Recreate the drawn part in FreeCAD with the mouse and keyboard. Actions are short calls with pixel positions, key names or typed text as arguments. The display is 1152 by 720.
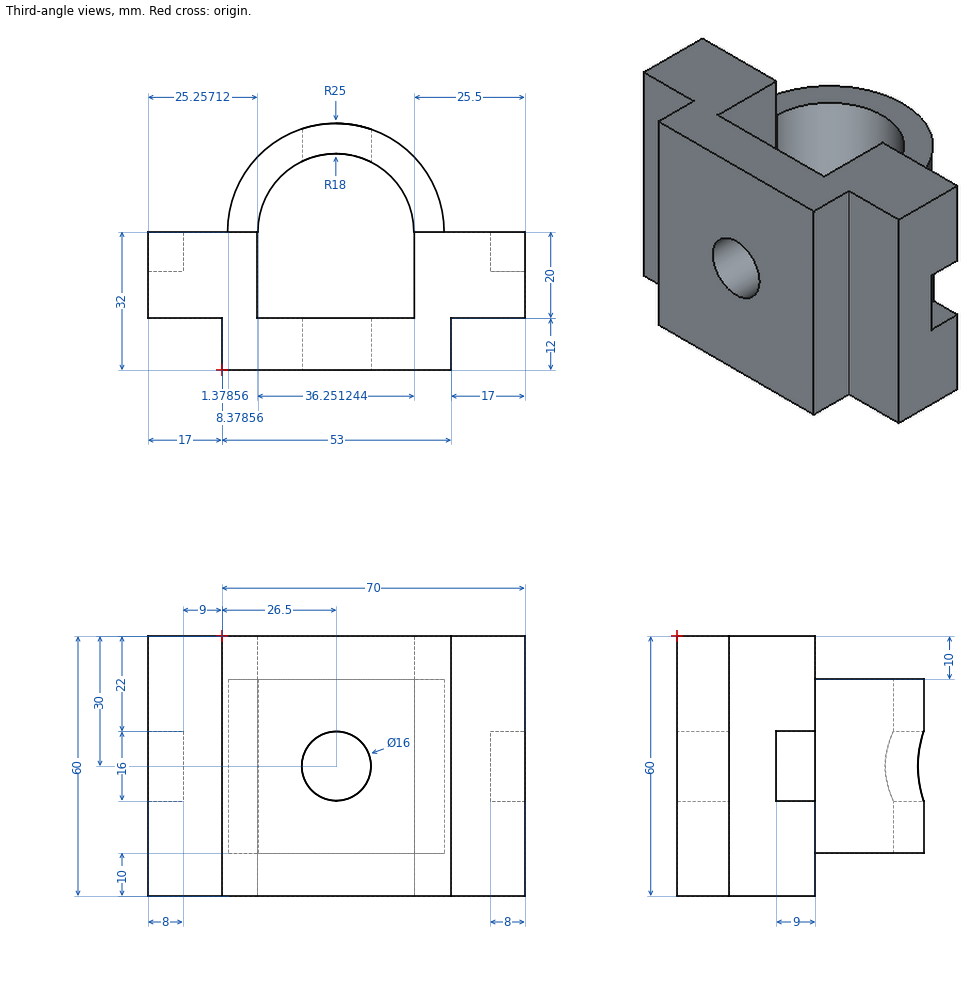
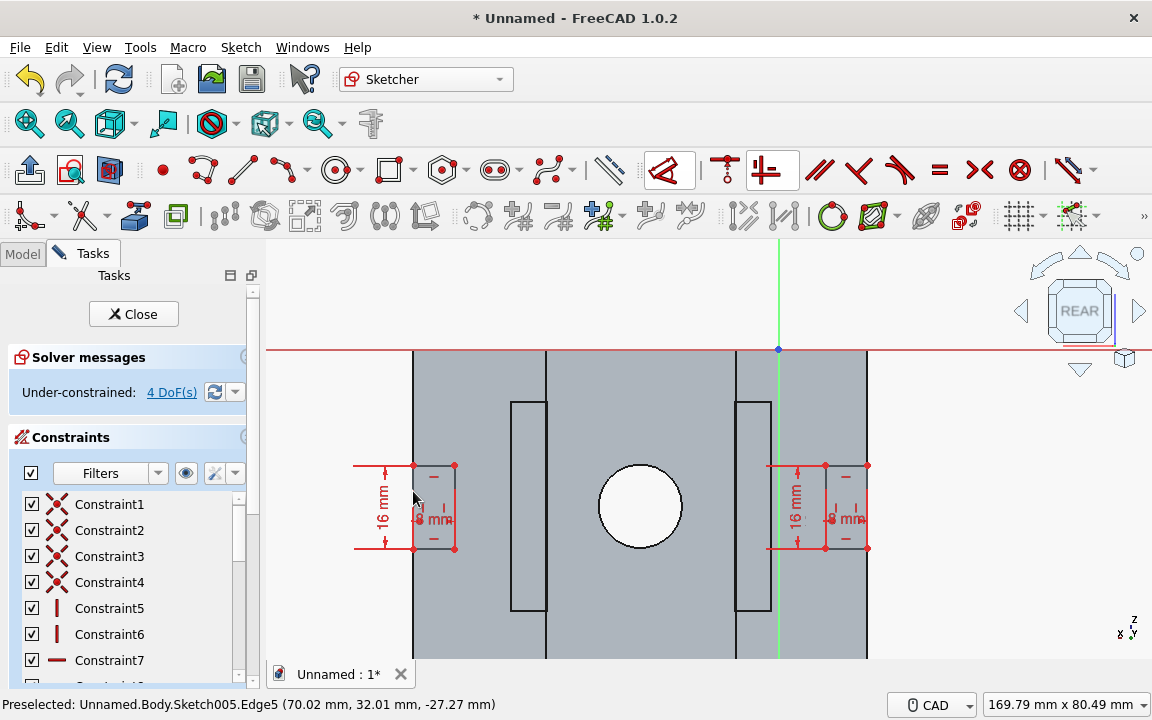
click(826, 466)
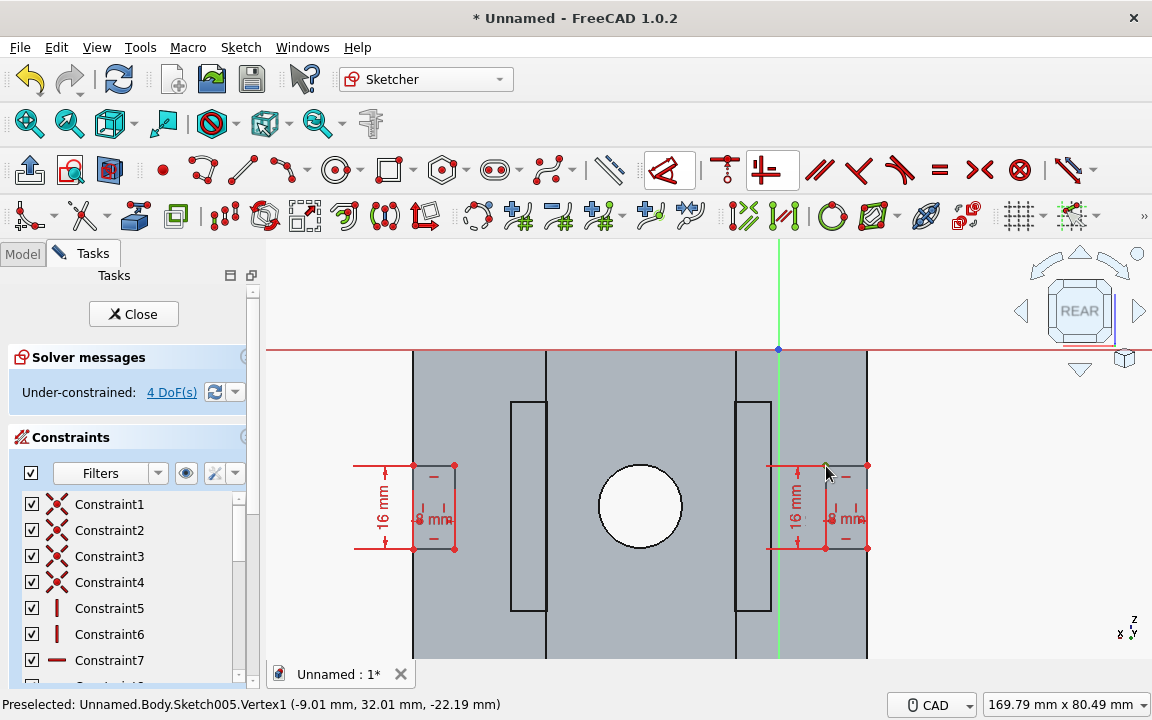
click(690, 170)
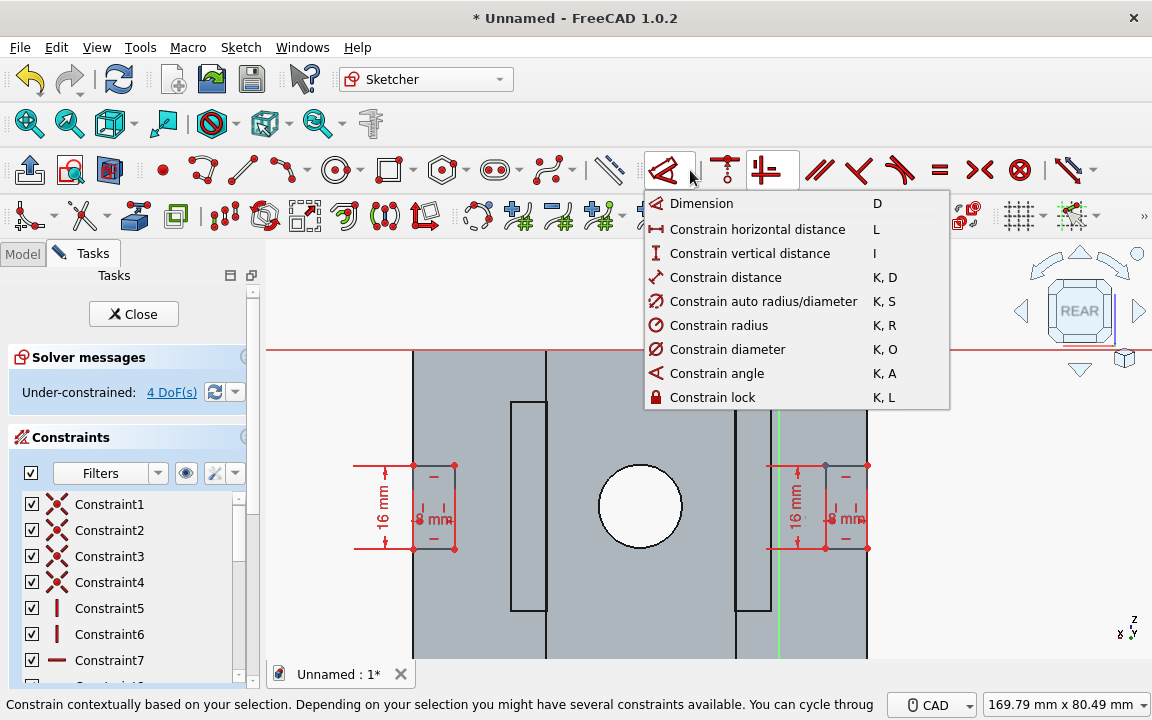
click(797, 229)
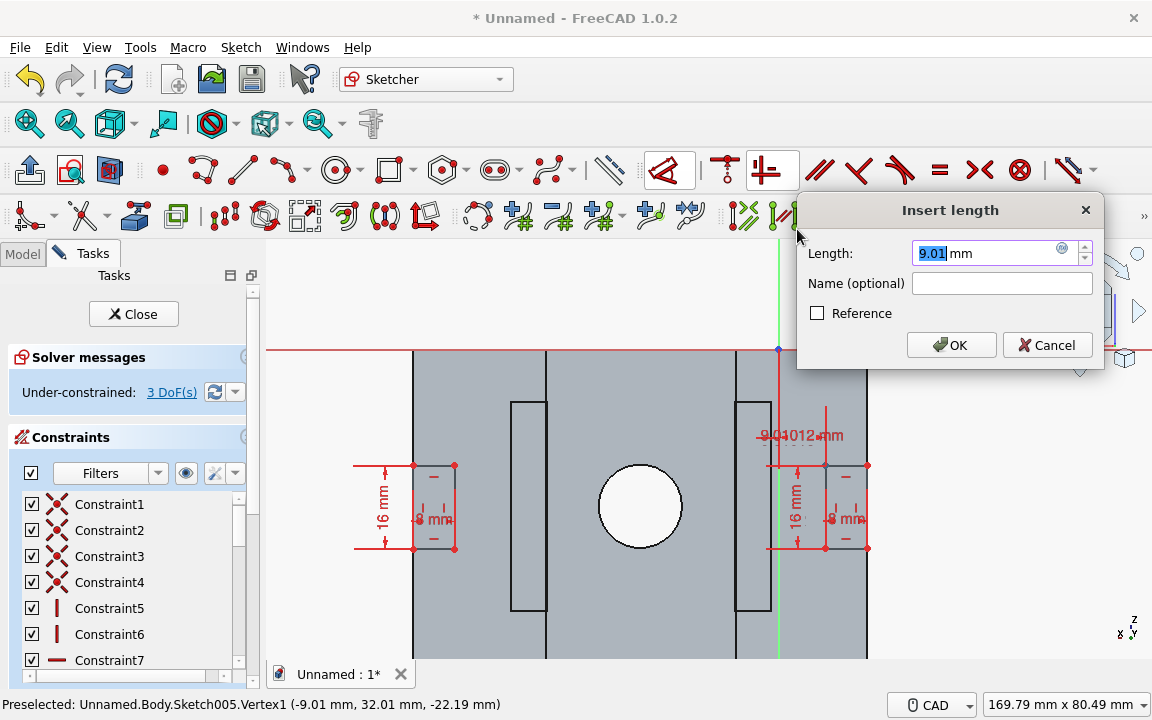
text(9)
key(Return)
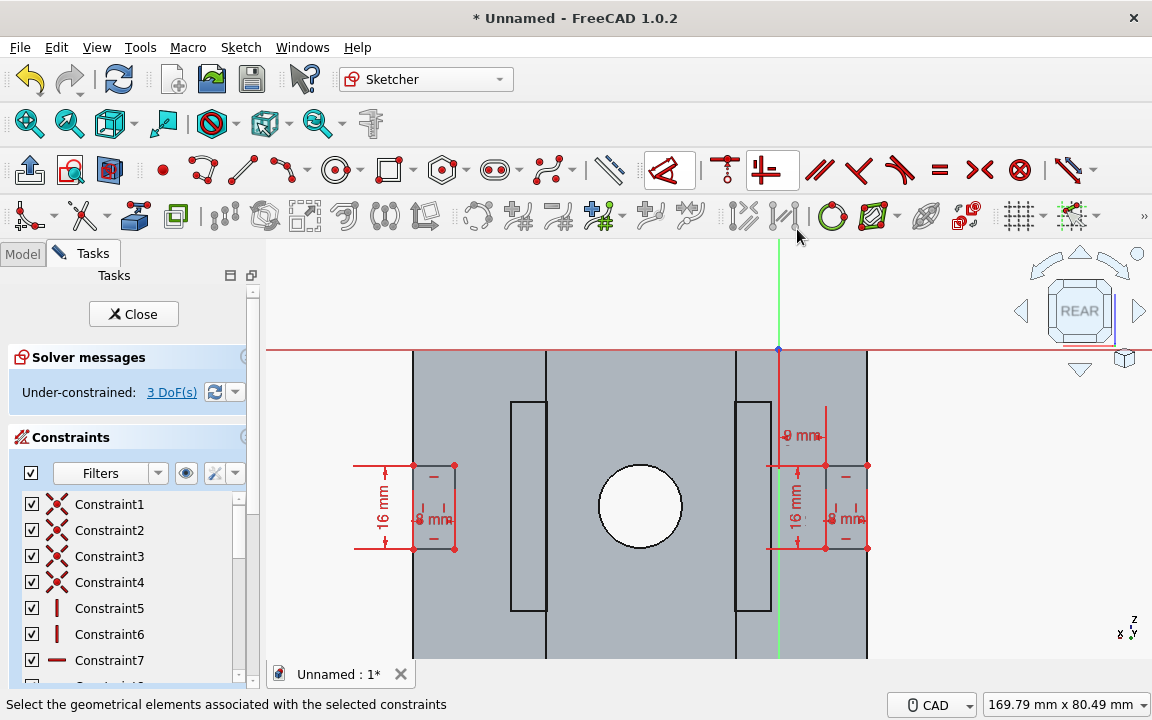
click(826, 466)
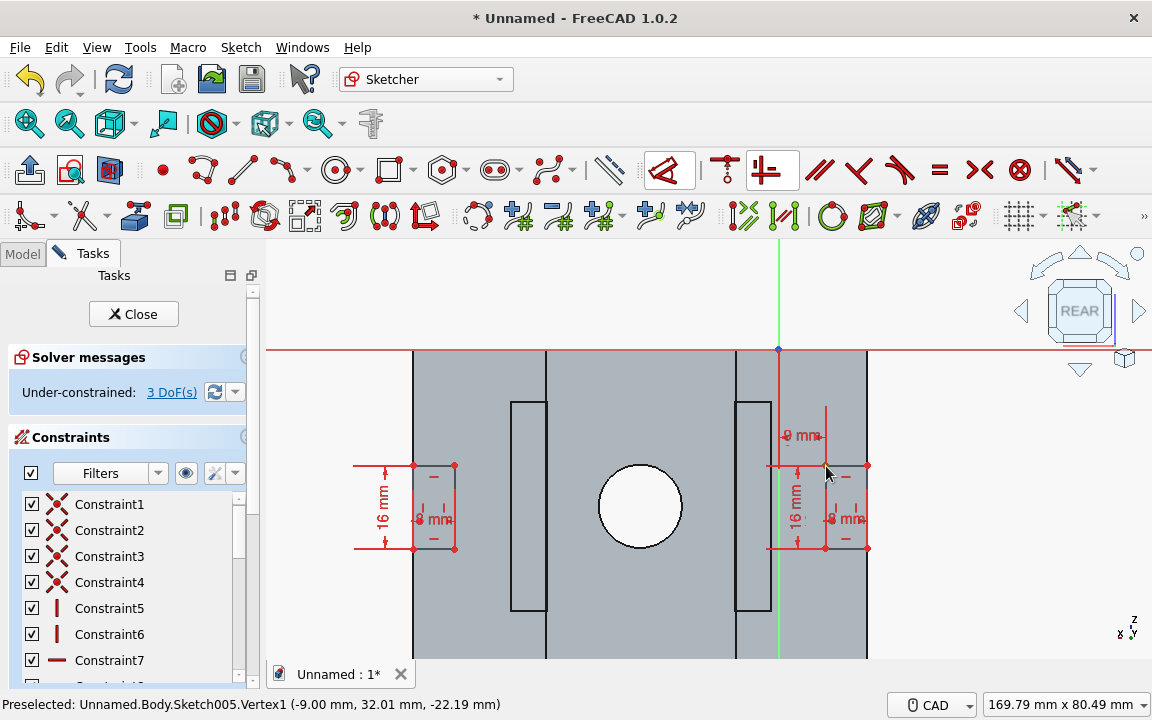
key(i)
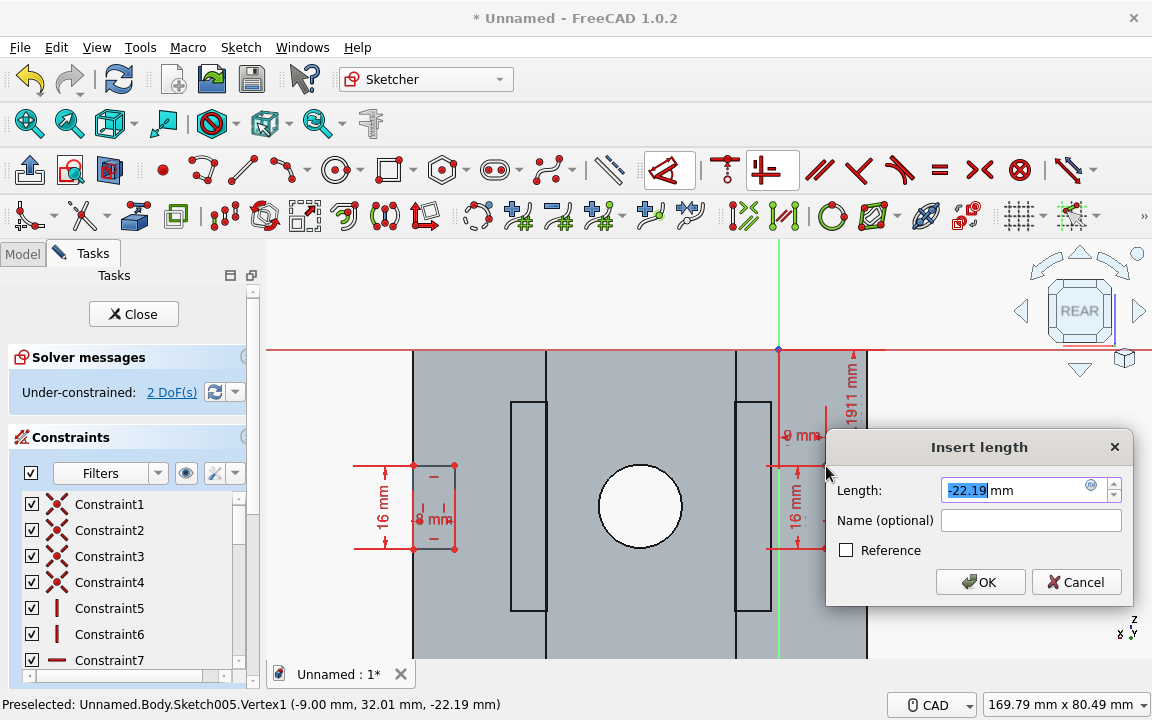
text(-22)
key(Return)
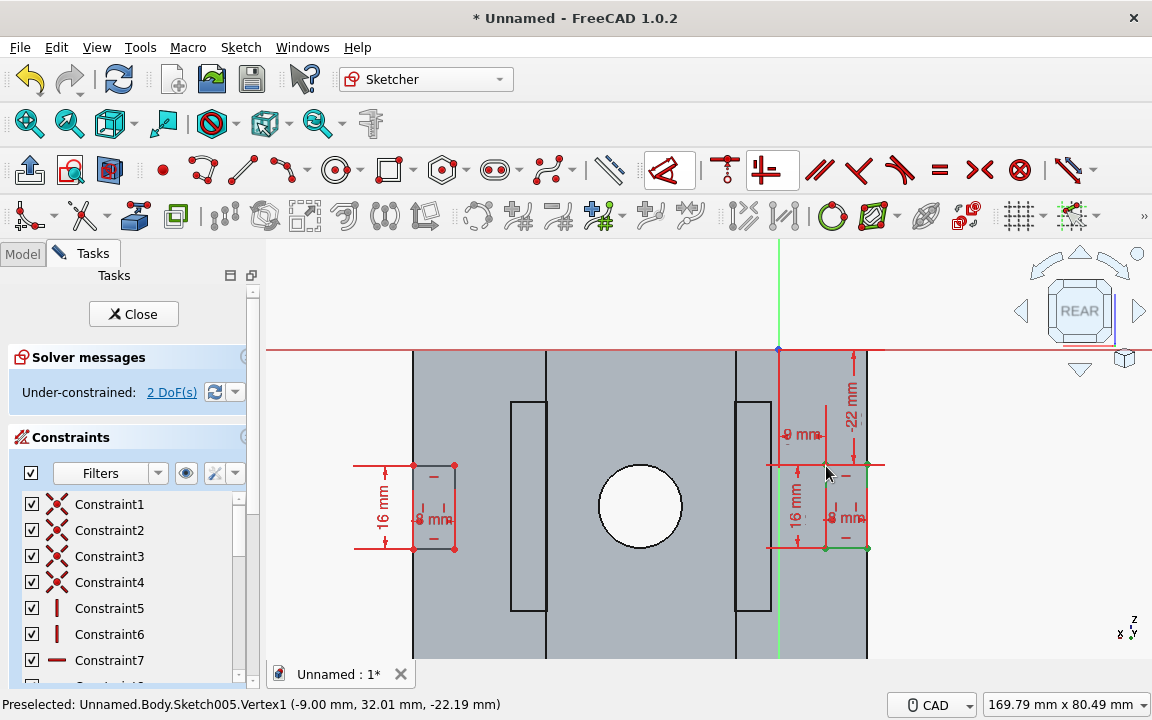
click(413, 466)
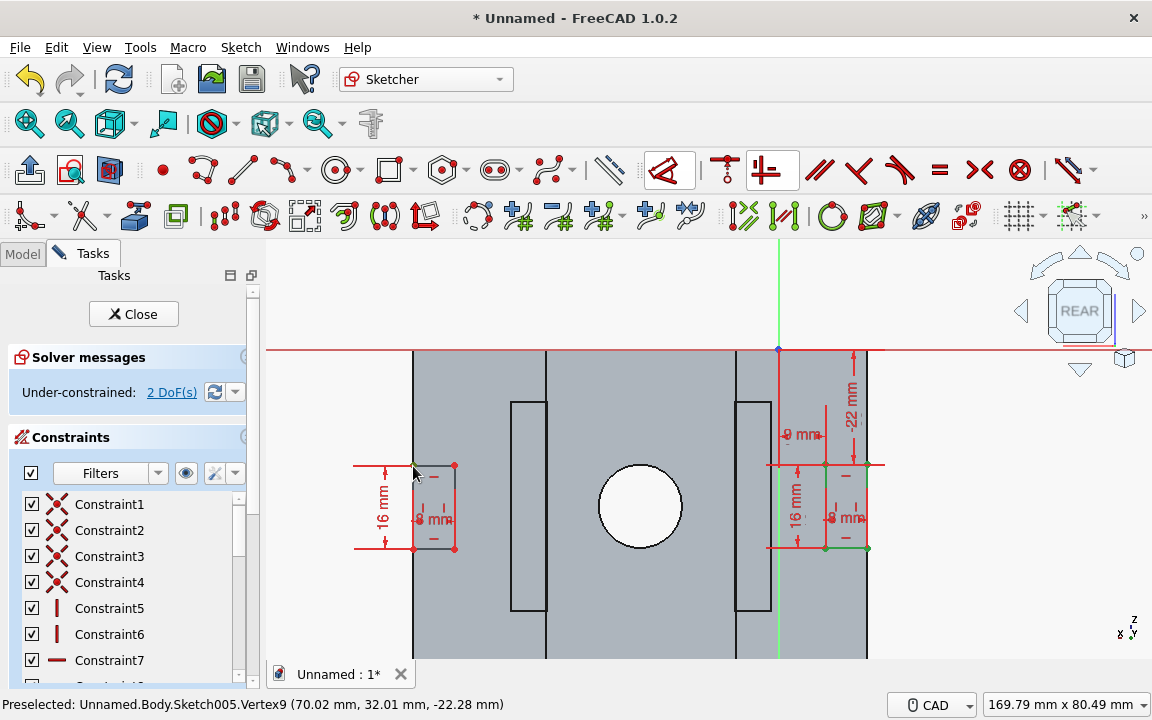
click(690, 170)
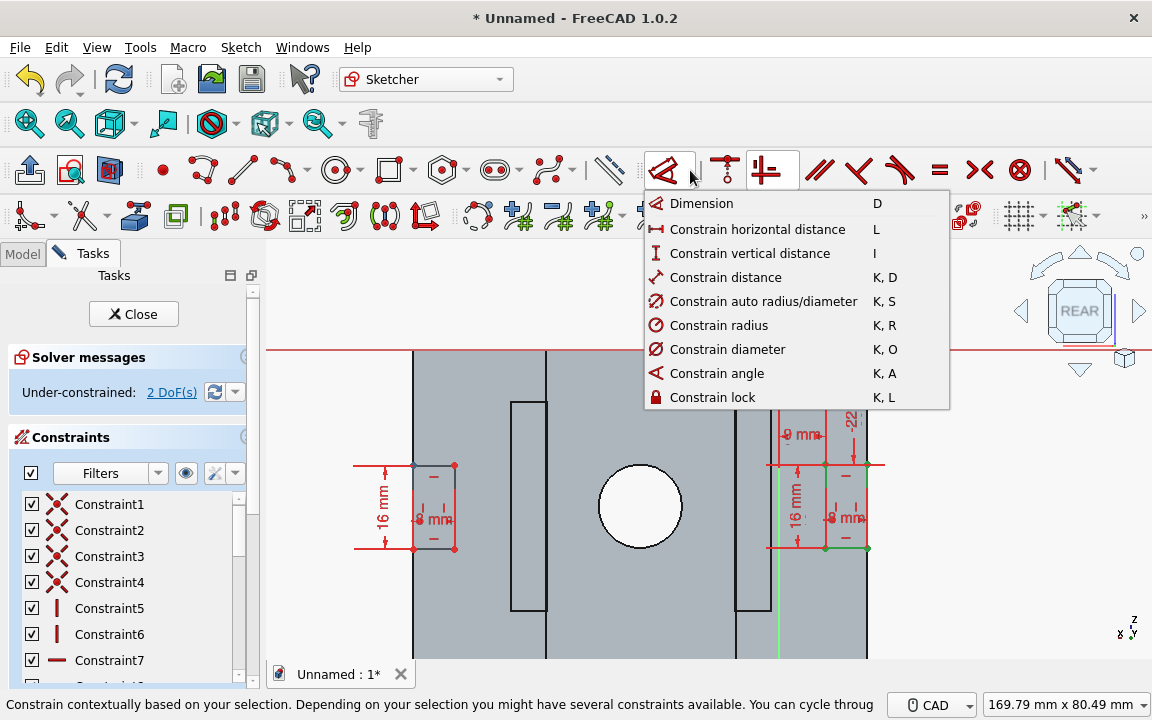
click(797, 229)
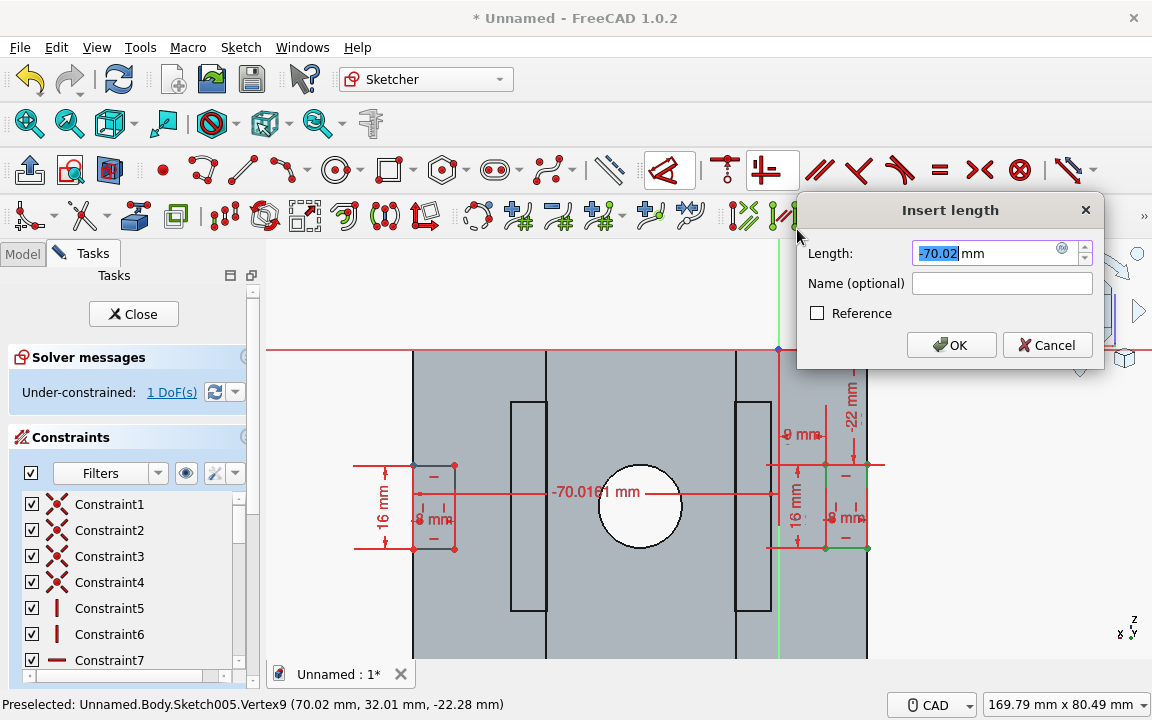
text(-70)
key(Return)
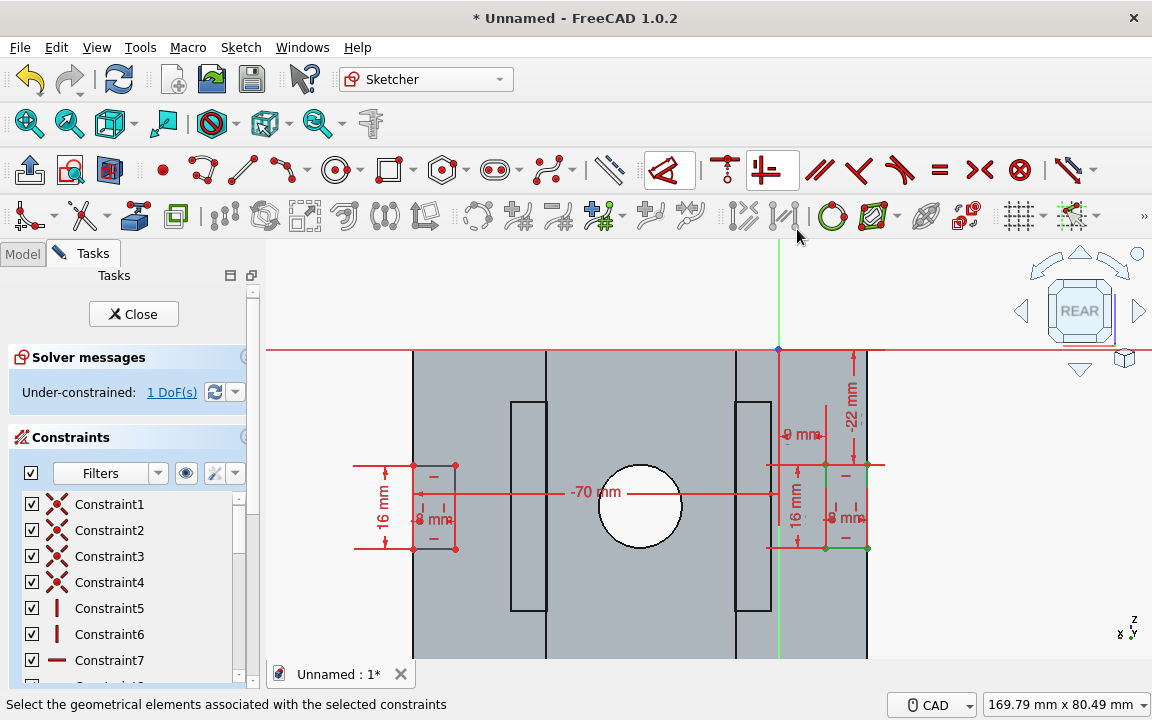
click(413, 466)